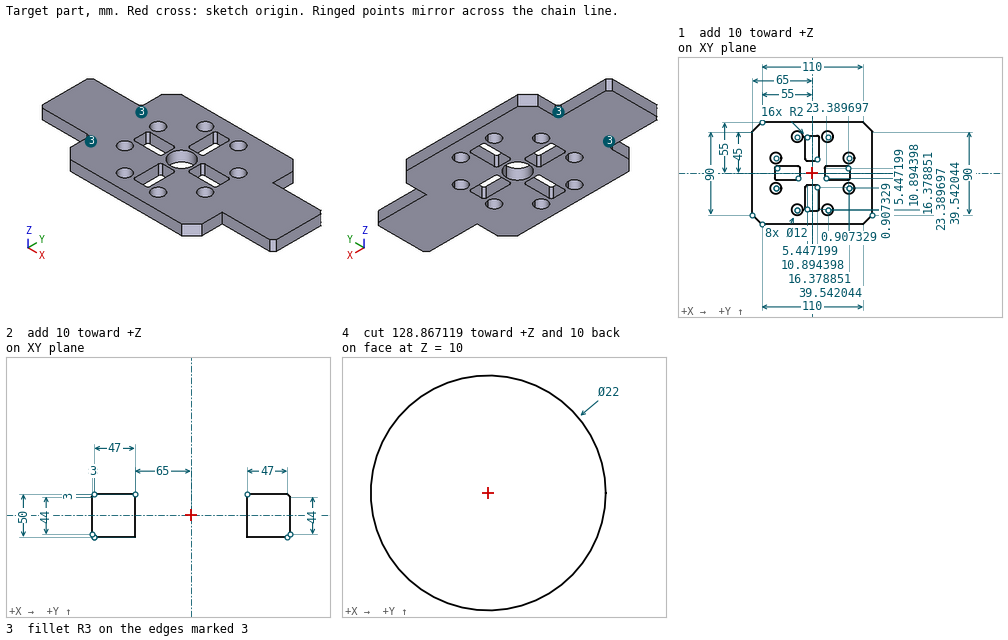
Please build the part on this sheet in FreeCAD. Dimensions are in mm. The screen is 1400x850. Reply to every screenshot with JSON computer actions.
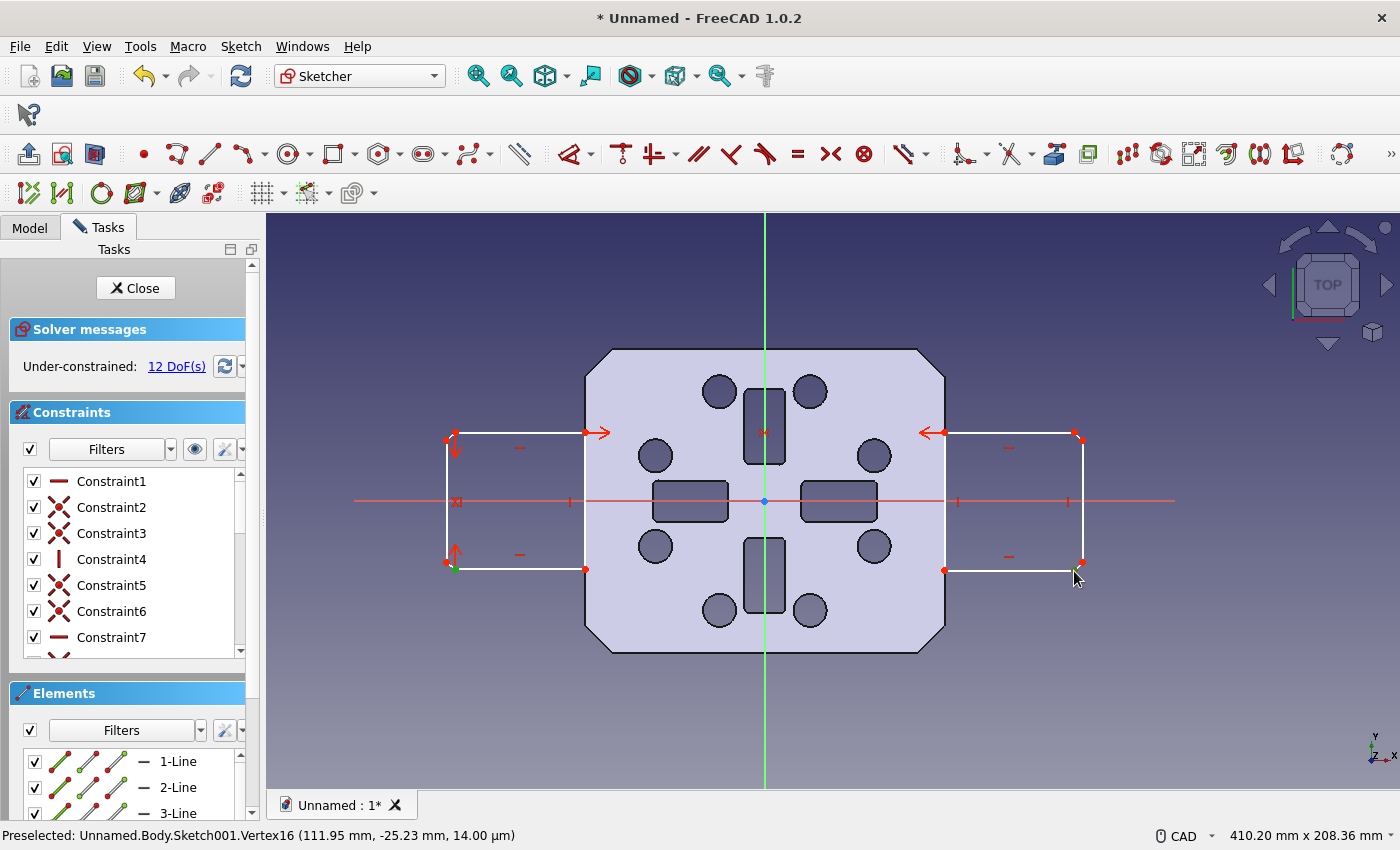
{"action": "left_click", "coordinate": [765, 724]}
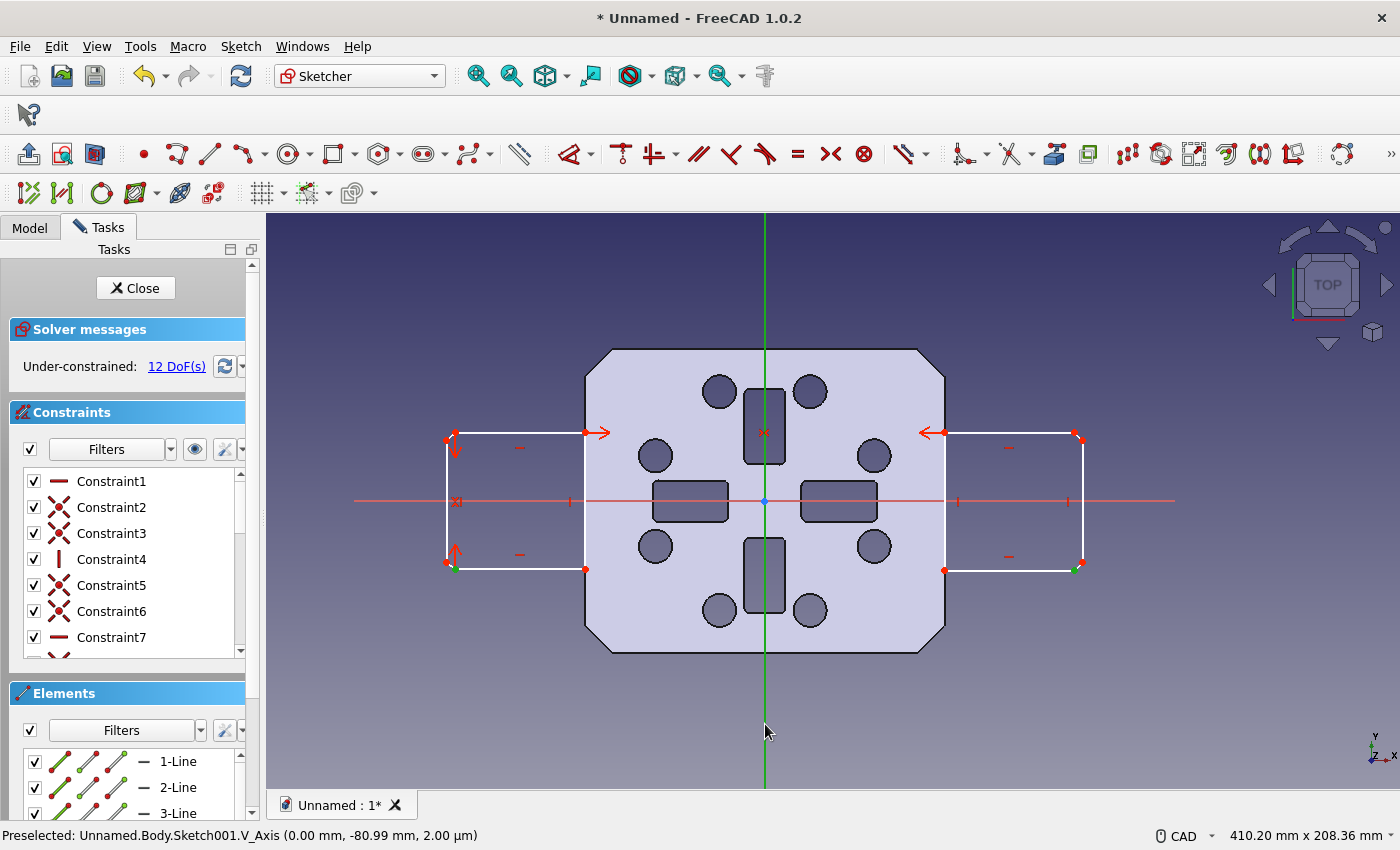
{"action": "left_click", "coordinate": [831, 154]}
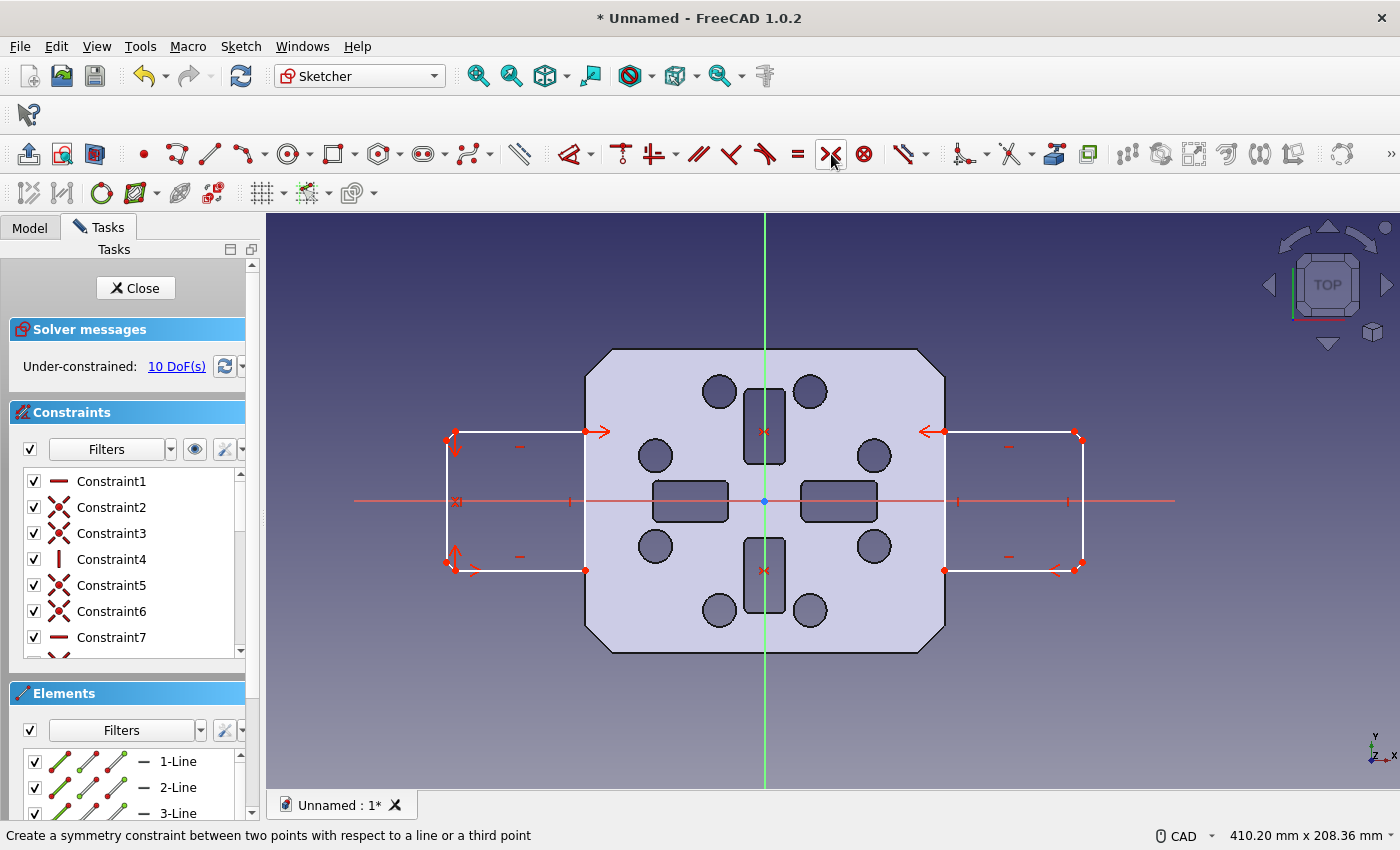
{"action": "left_click", "coordinate": [447, 563]}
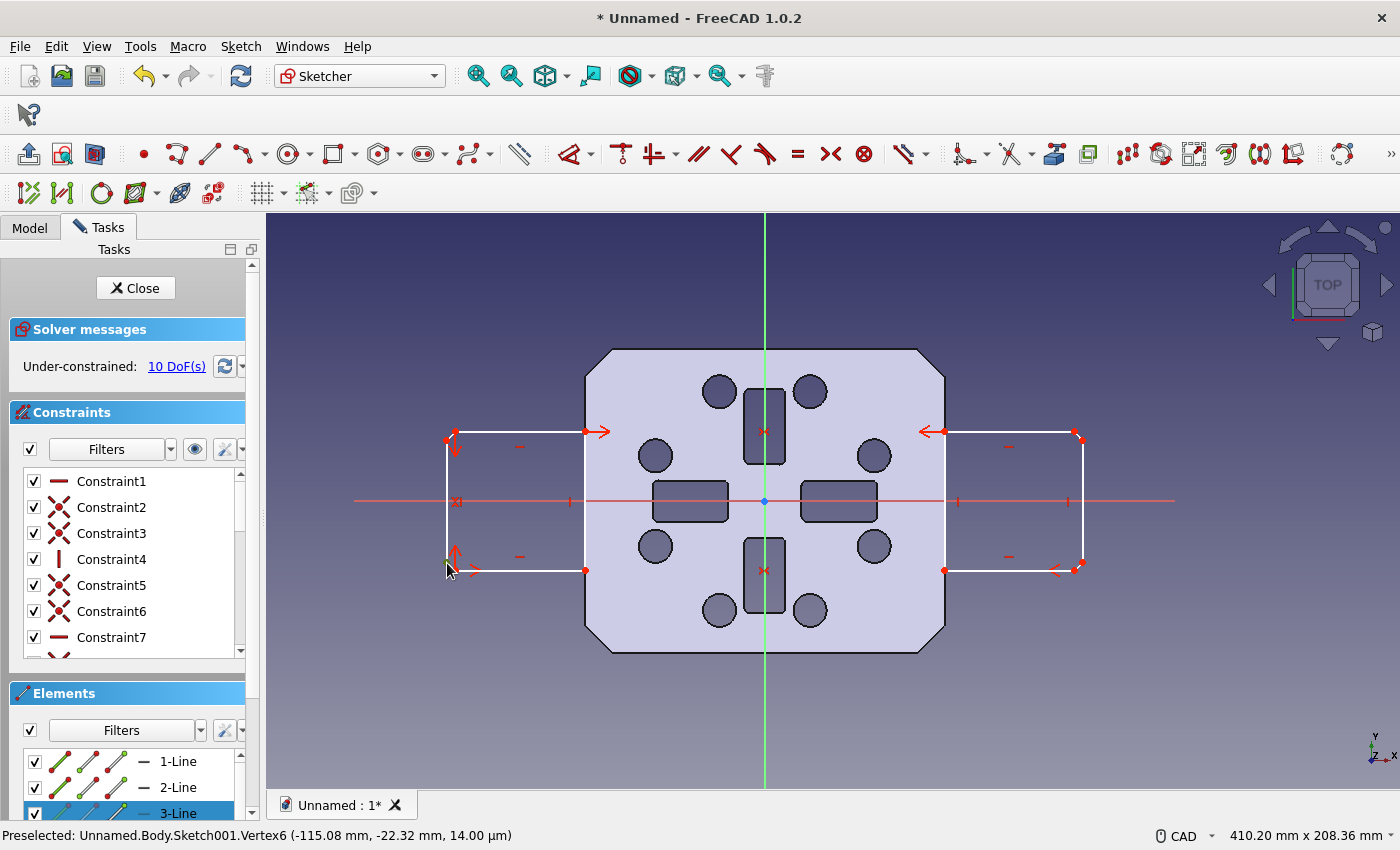
{"action": "left_click", "coordinate": [1083, 563]}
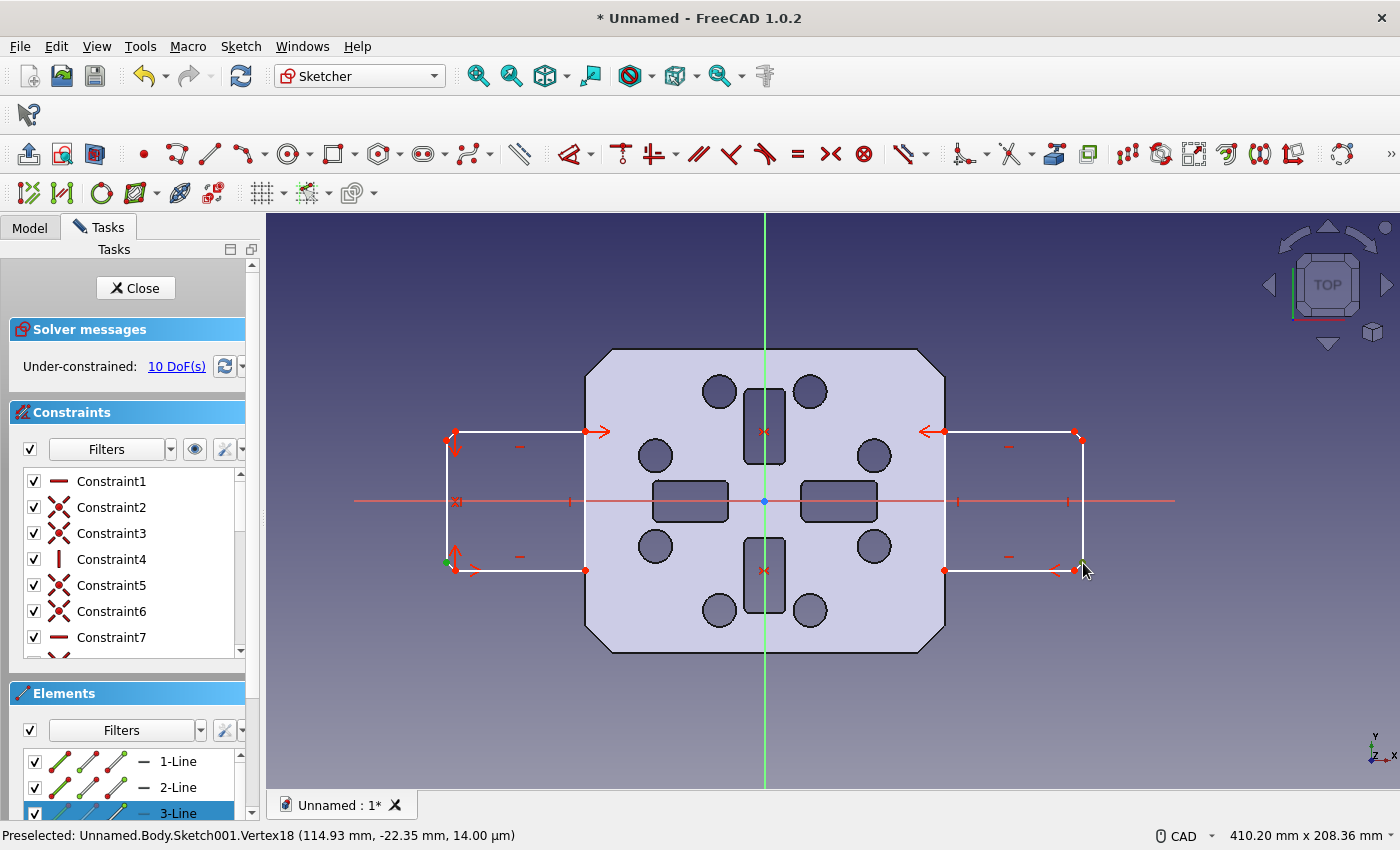
{"action": "left_click", "coordinate": [765, 724]}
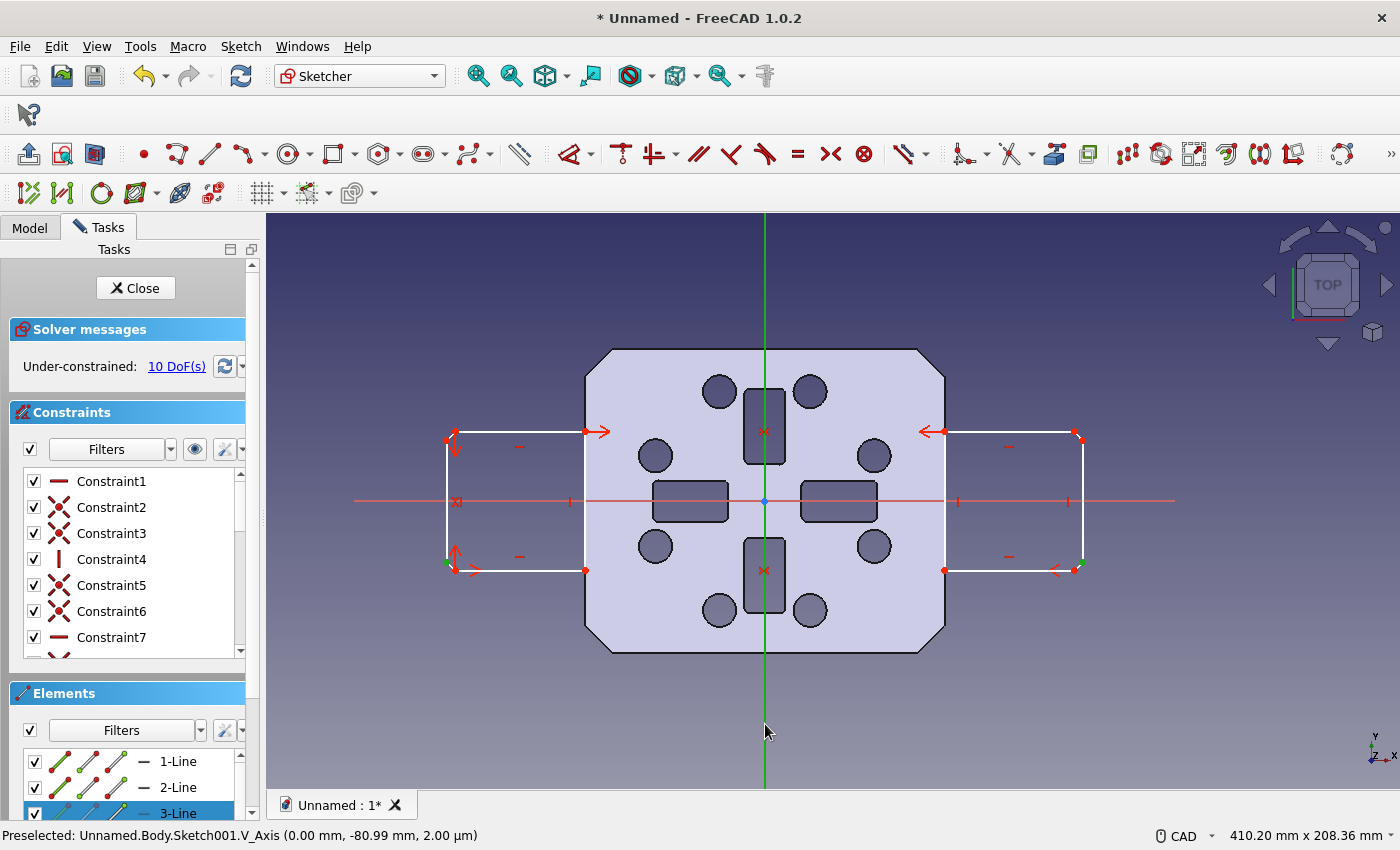
{"action": "left_click", "coordinate": [831, 154]}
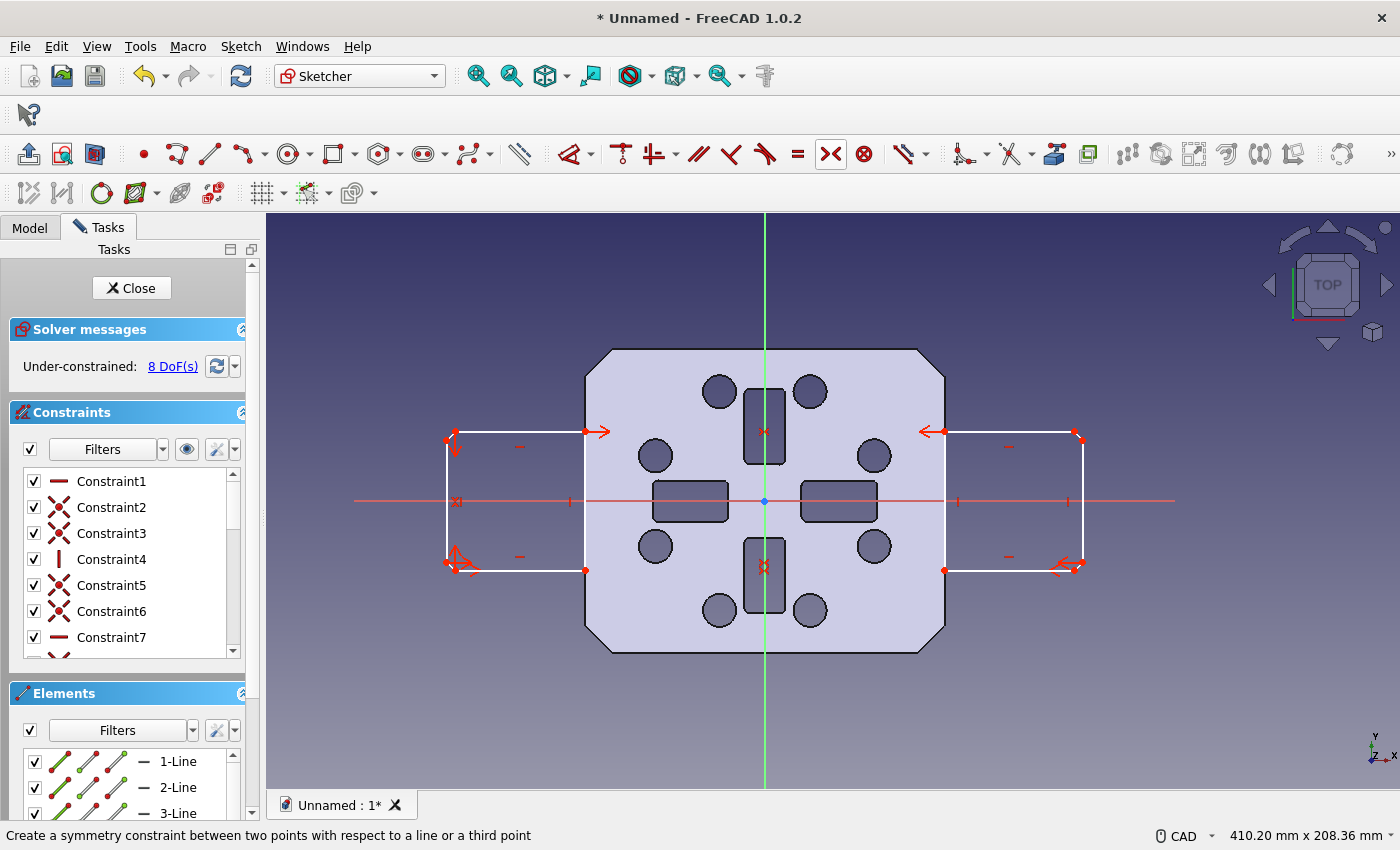
{"action": "left_click", "coordinate": [568, 154]}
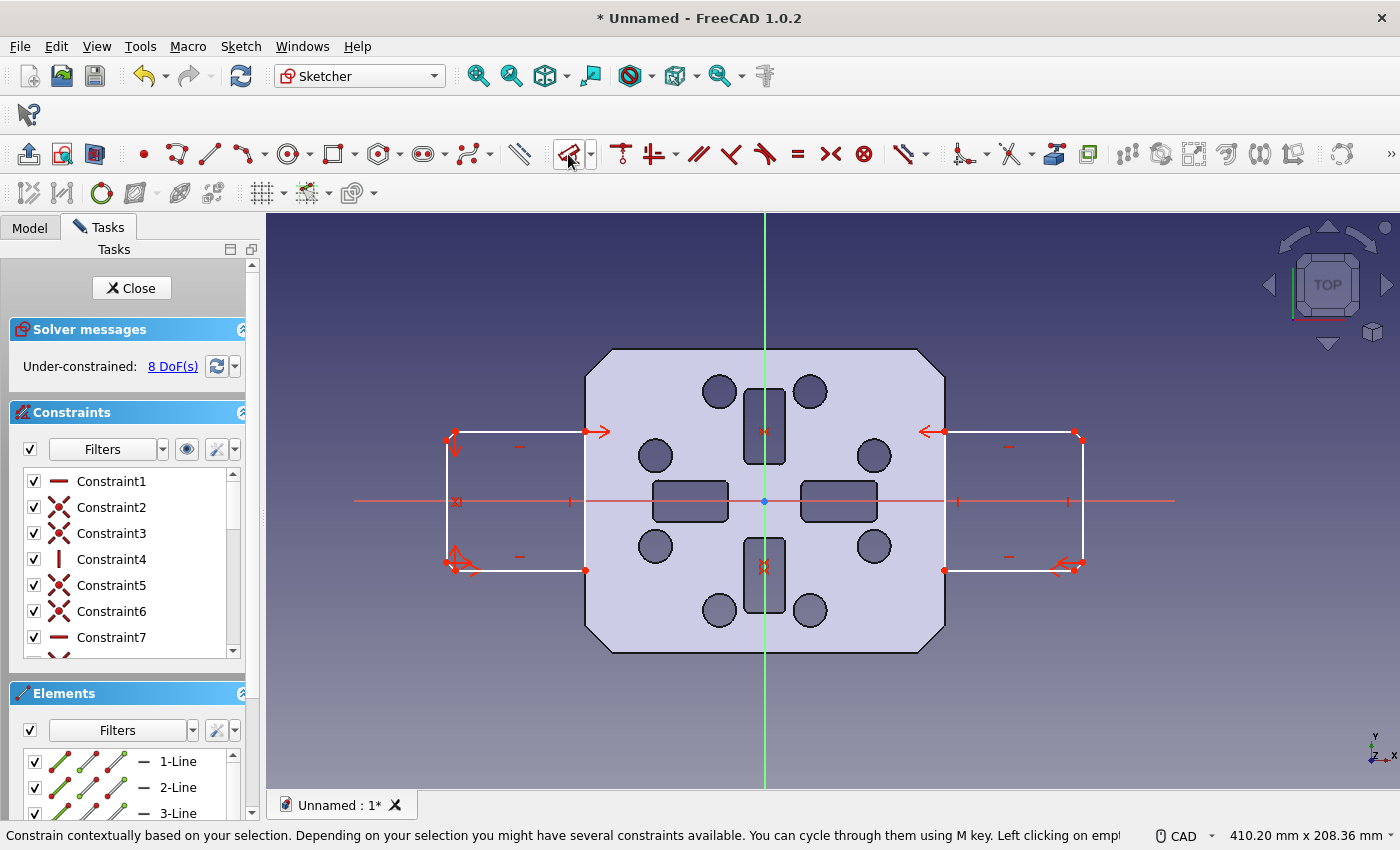
{"action": "left_click", "coordinate": [546, 432]}
{"action": "left_click", "coordinate": [520, 398]}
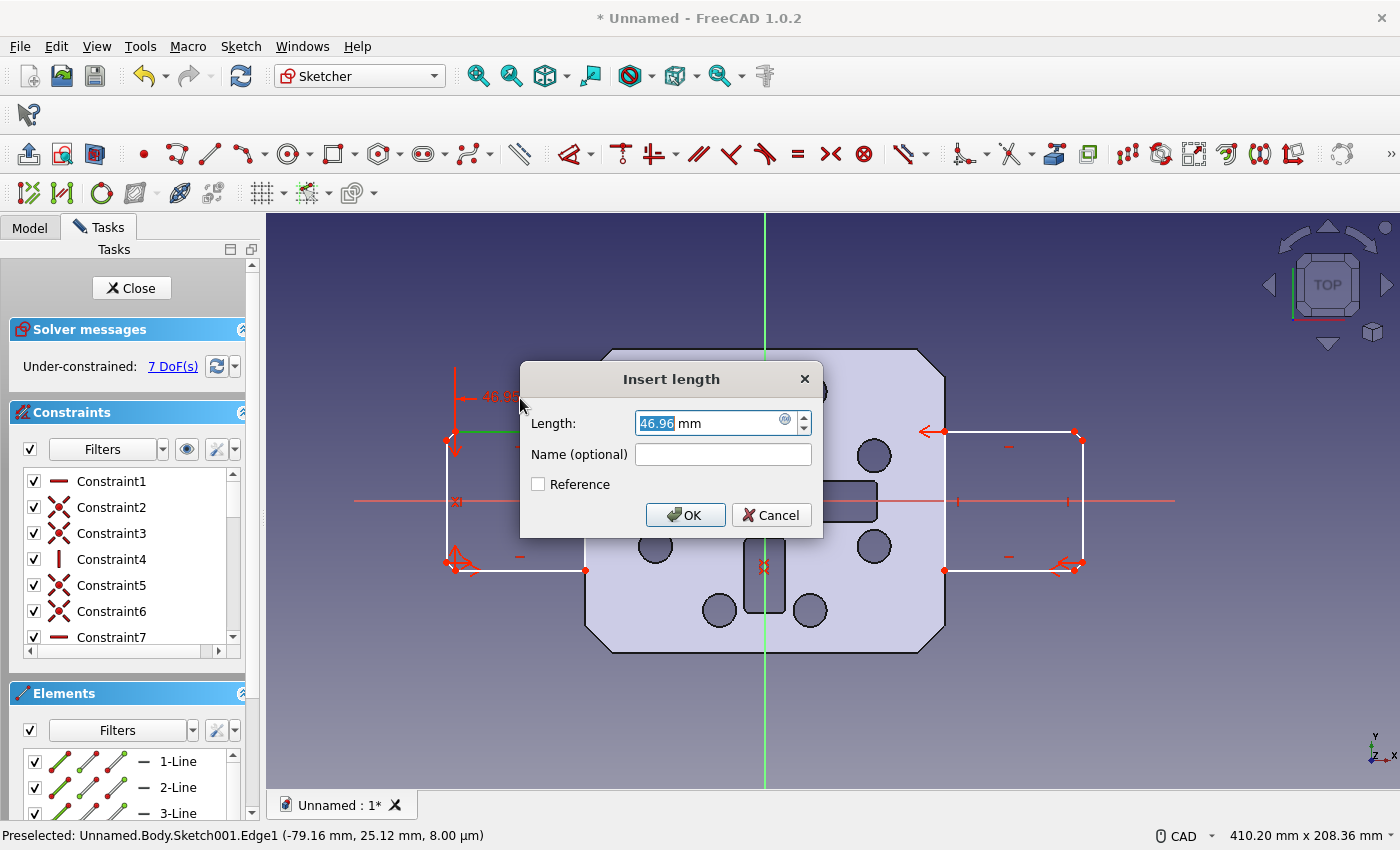
{"action": "type", "text": "47"}
{"action": "key", "text": "Return"}